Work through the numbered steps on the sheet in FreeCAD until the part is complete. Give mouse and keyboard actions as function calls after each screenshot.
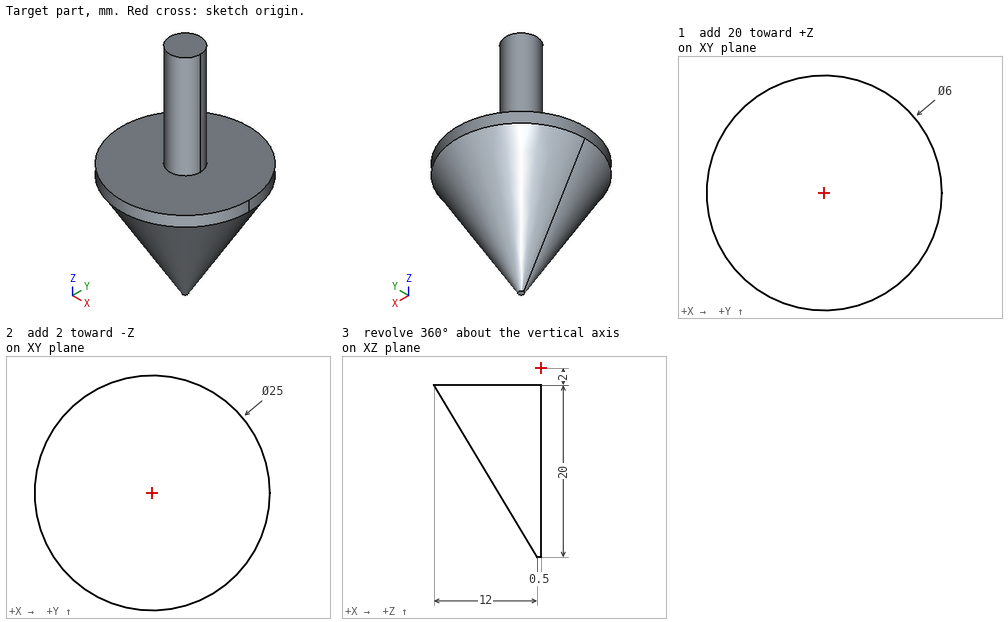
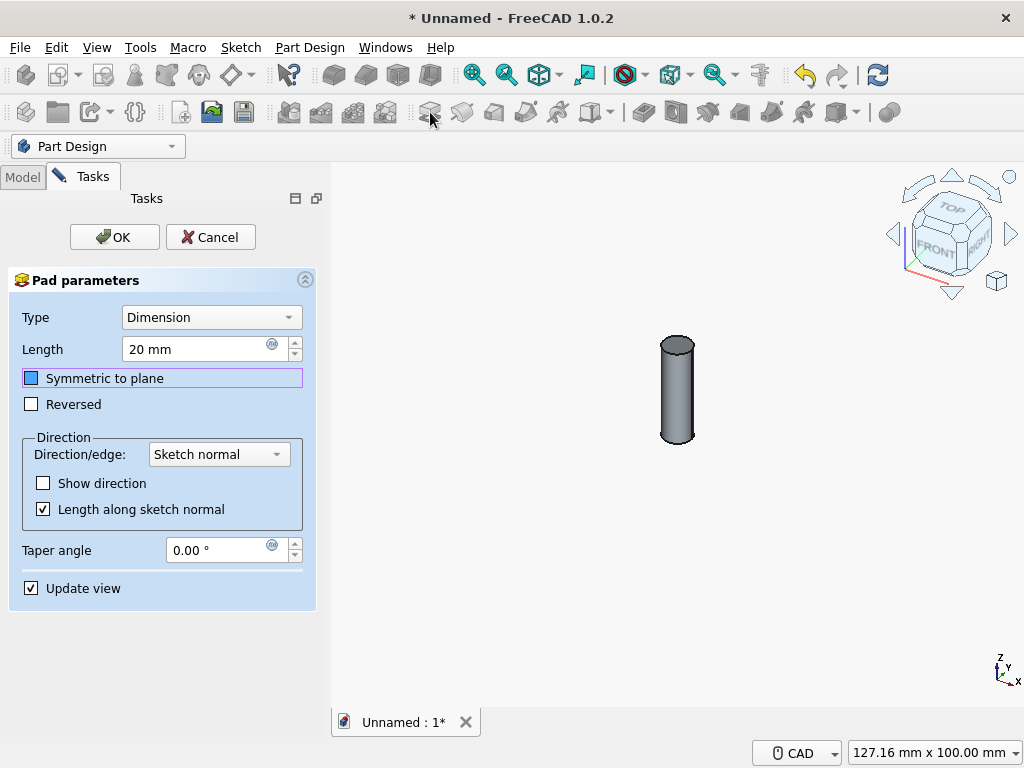
click(115, 237)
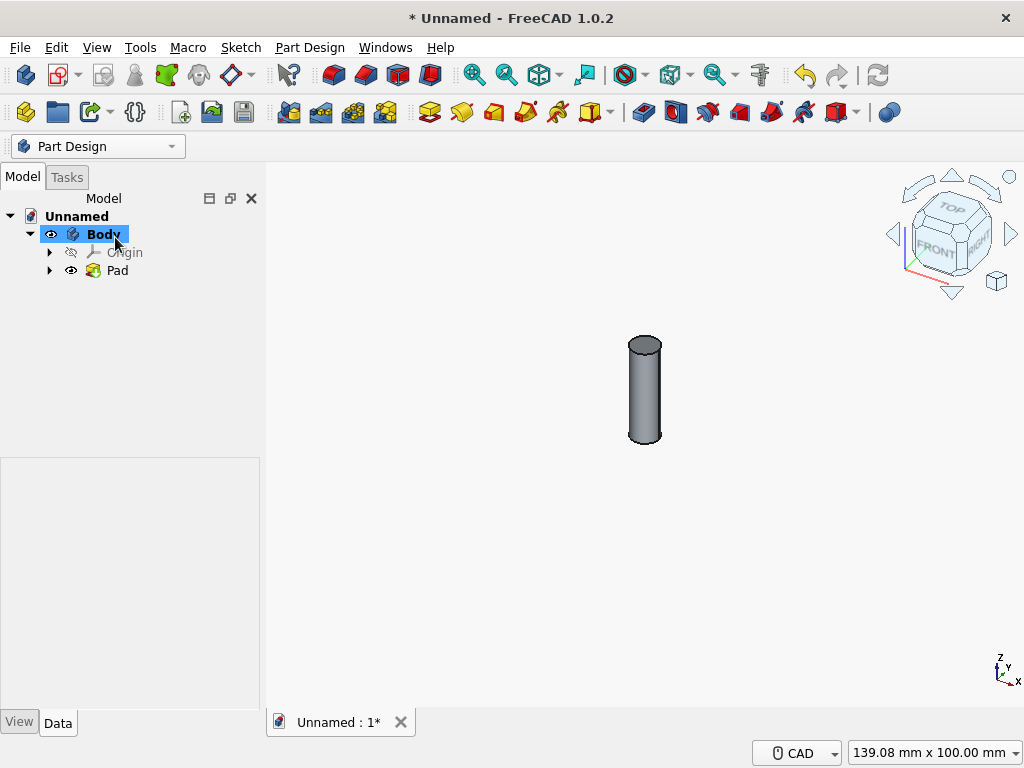
click(476, 76)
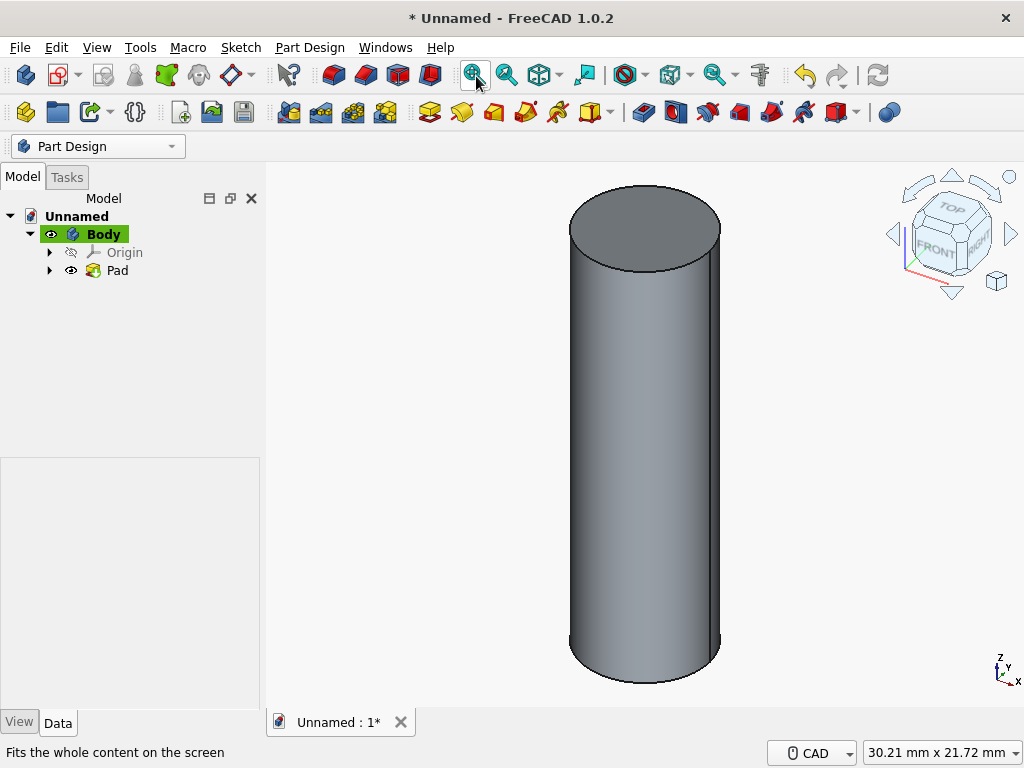
click(58, 76)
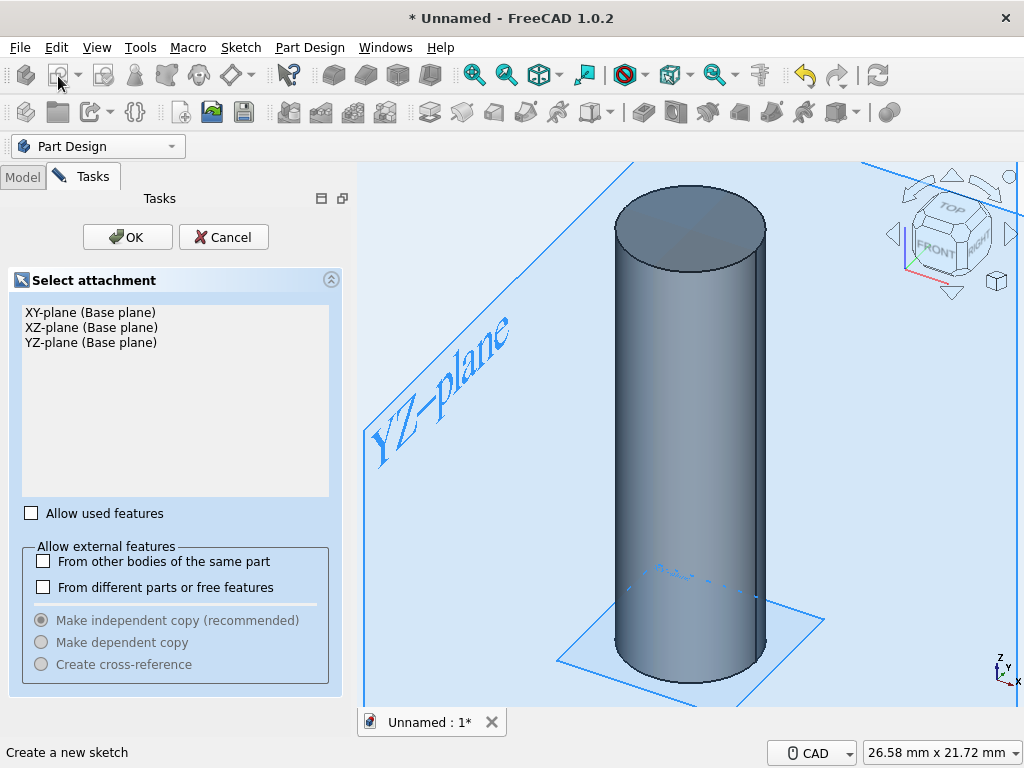
click(82, 312)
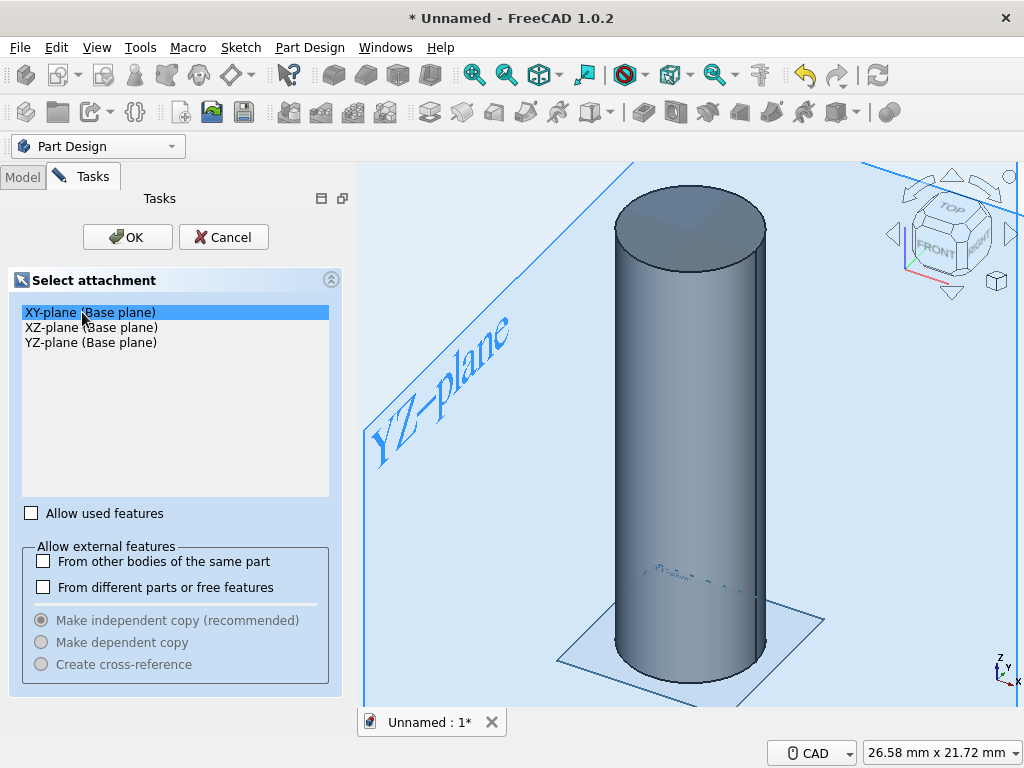
click(128, 237)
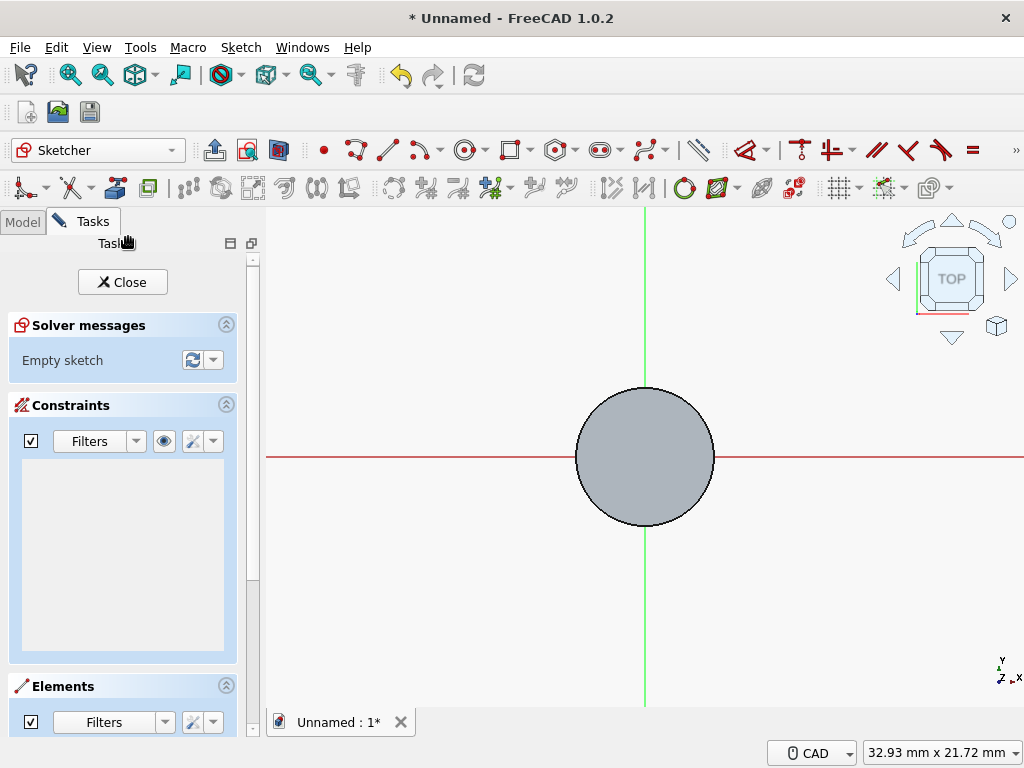
click(280, 150)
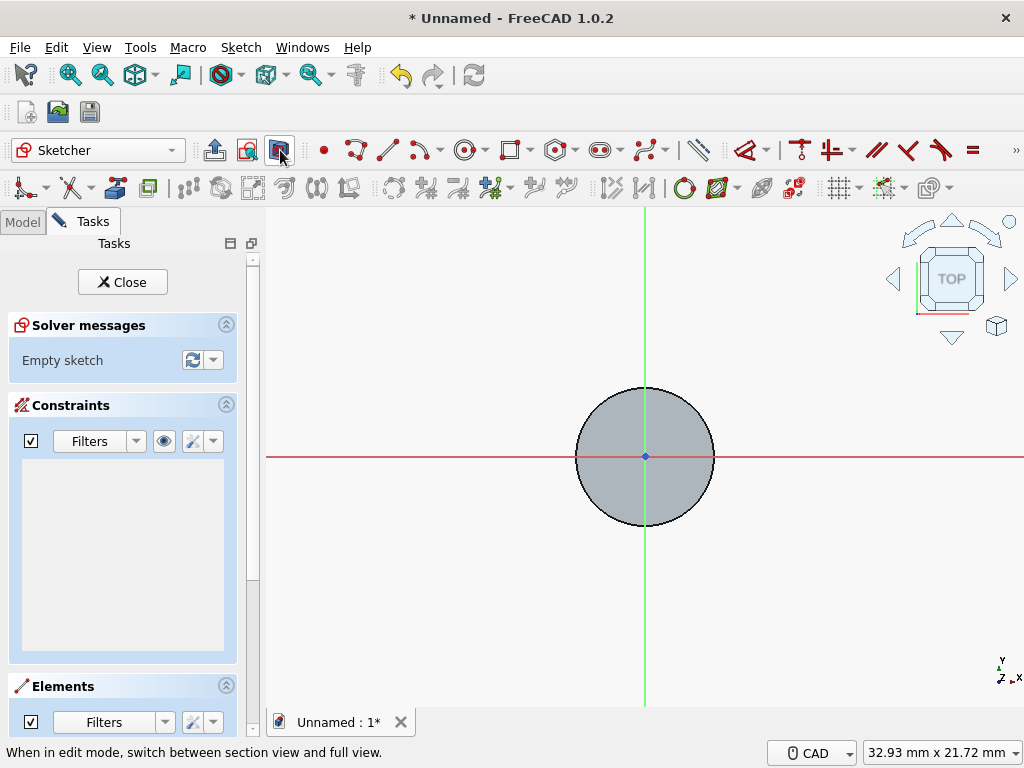
scroll(493, 457, down, 3)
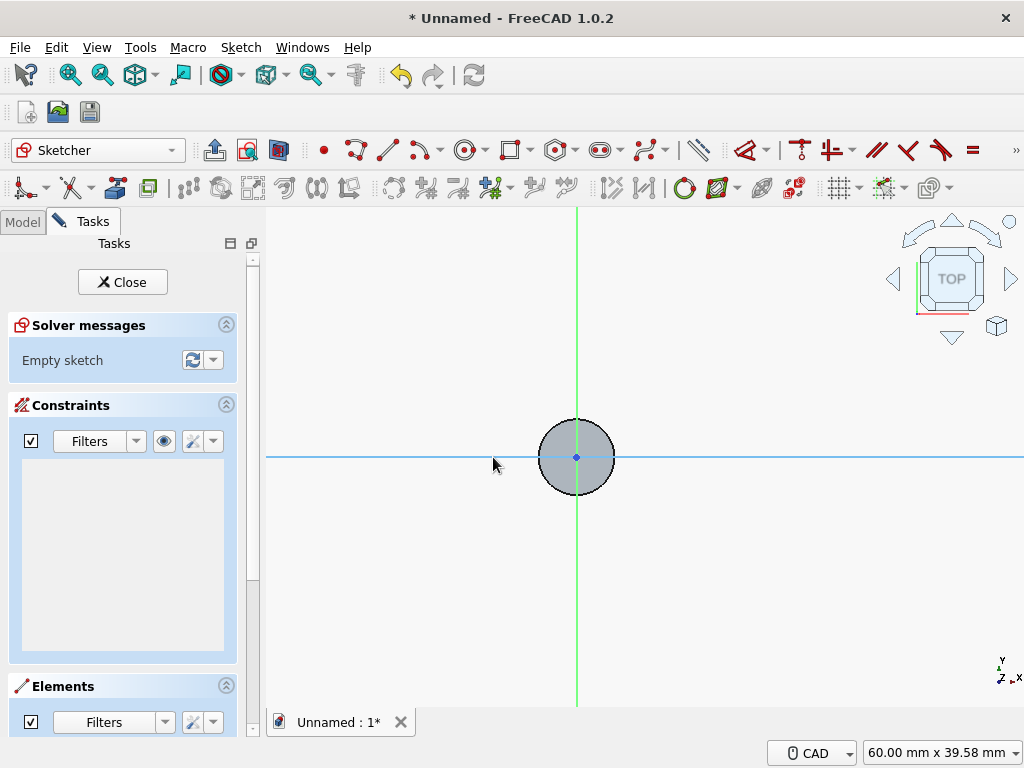
click(466, 150)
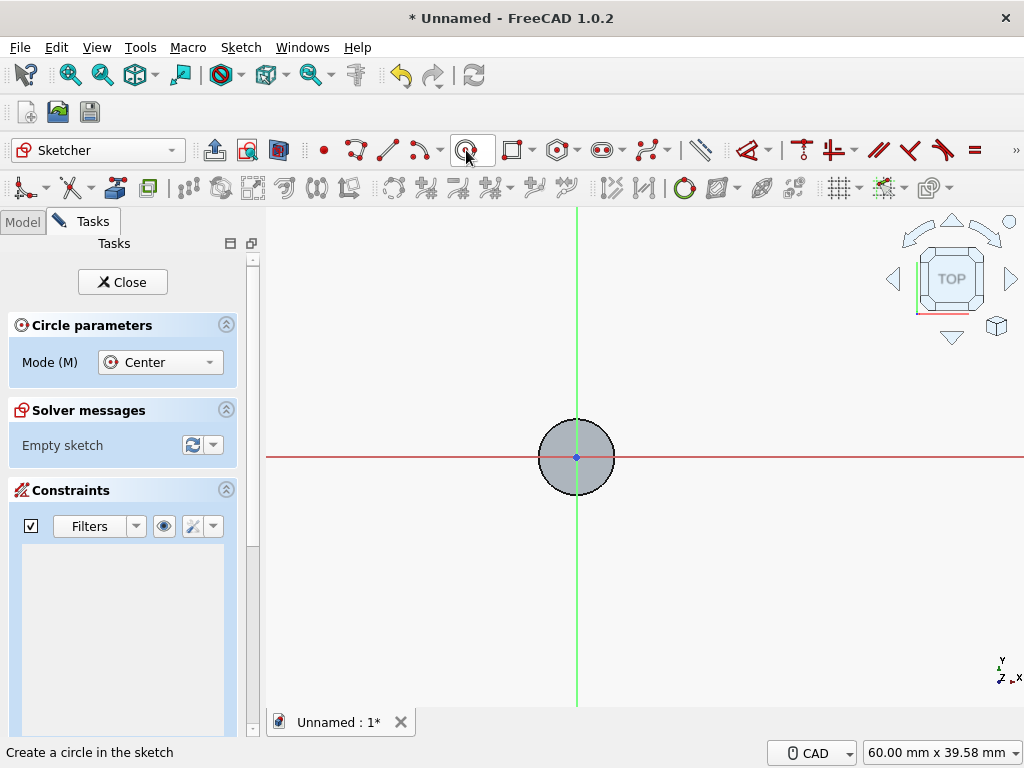
click(577, 457)
click(688, 346)
key(Escape)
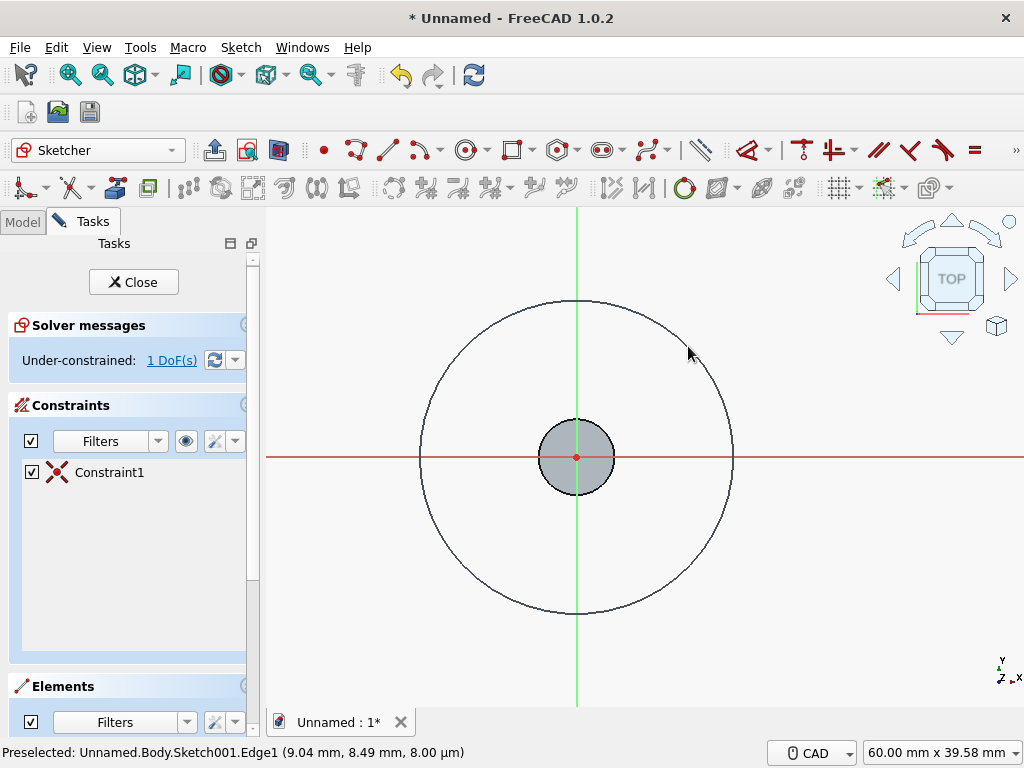
click(748, 150)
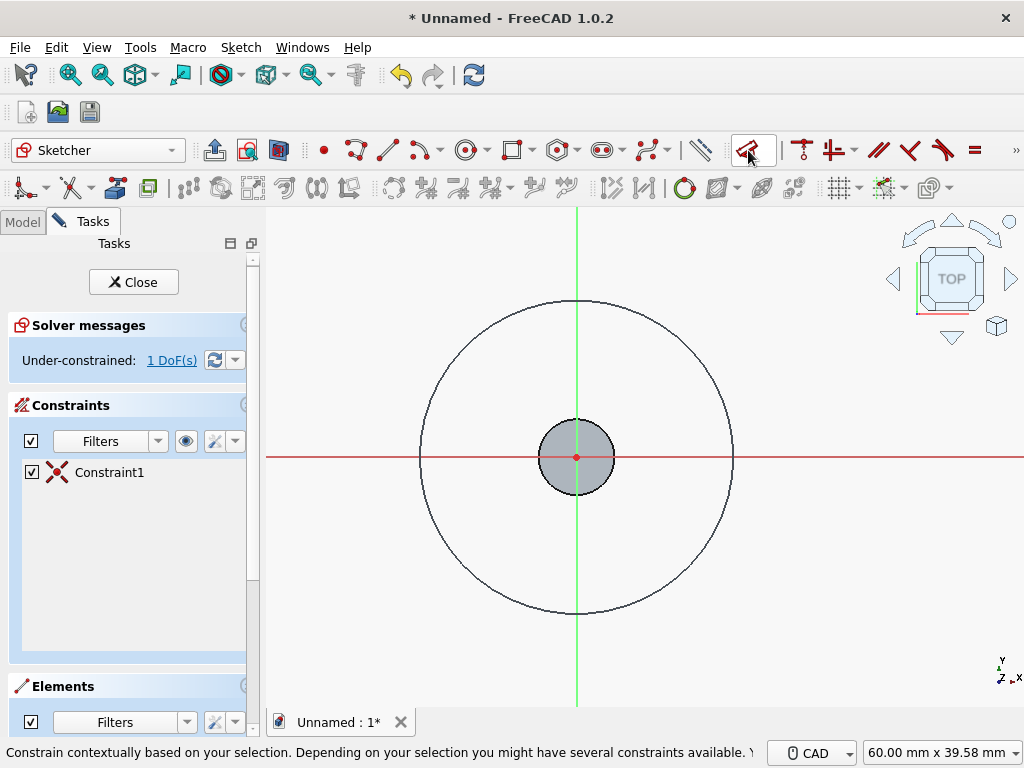
click(687, 346)
click(710, 323)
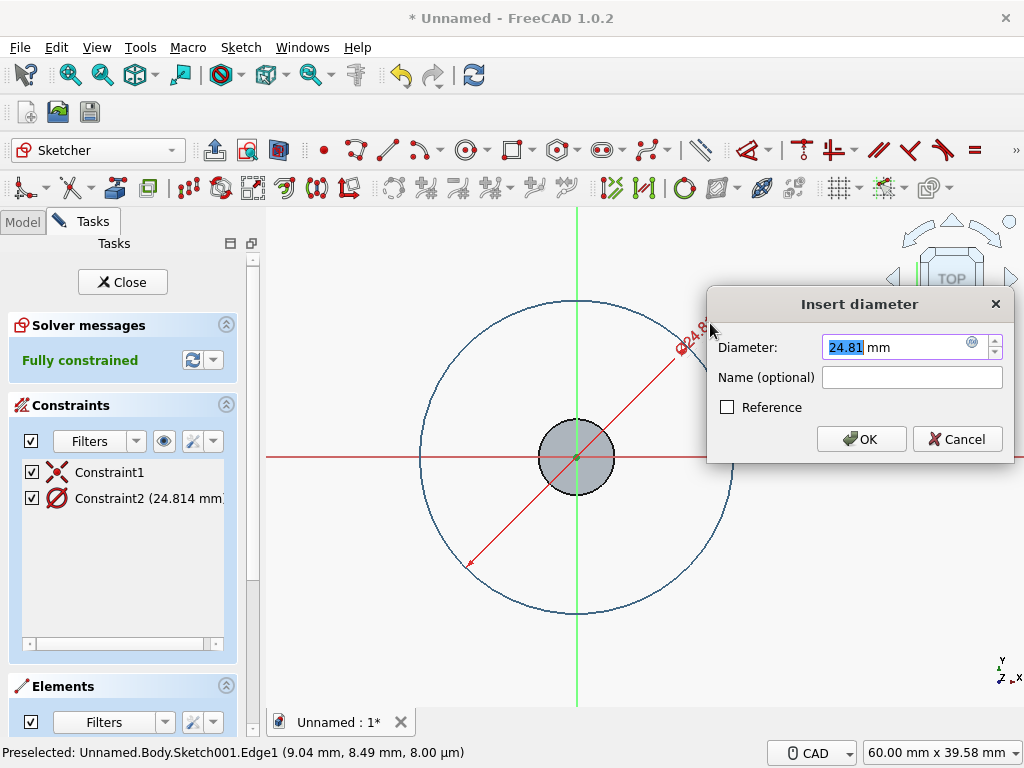
text(25)
key(Return)
key(Escape)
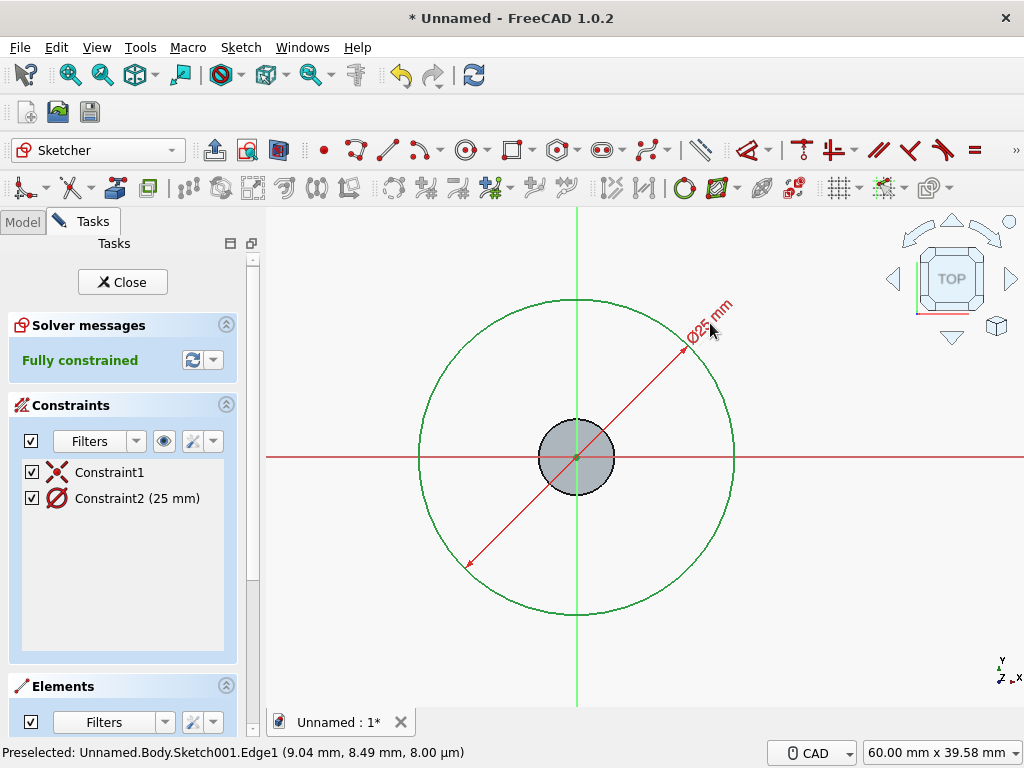
click(123, 282)